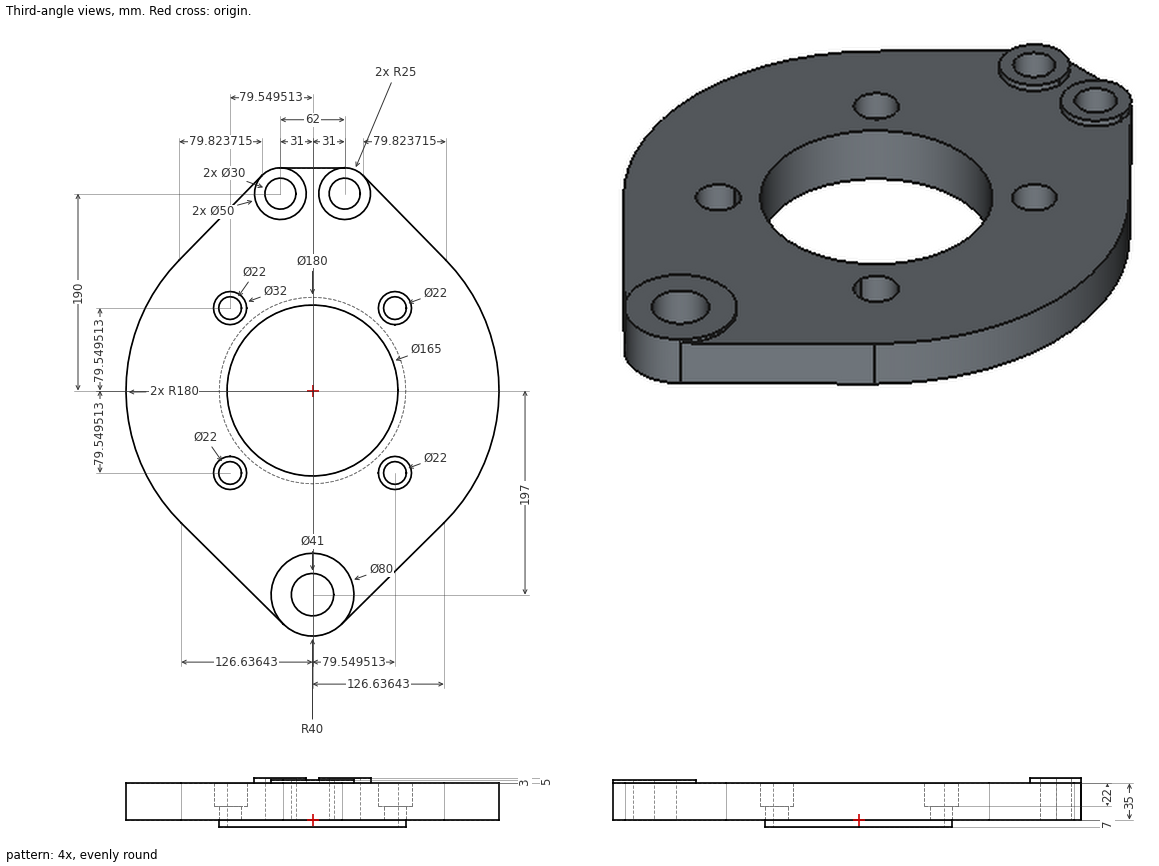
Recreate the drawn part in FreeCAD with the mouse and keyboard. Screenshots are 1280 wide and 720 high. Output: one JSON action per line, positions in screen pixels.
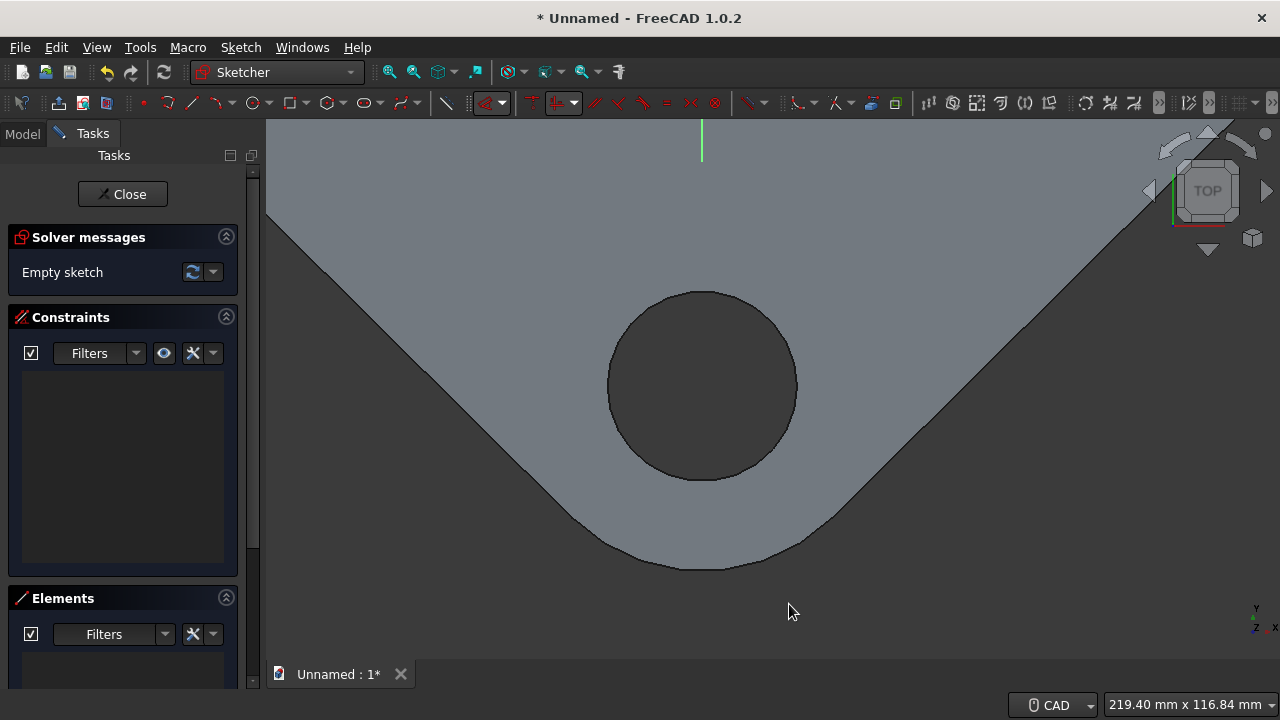
{"action": "key", "text": "g c"}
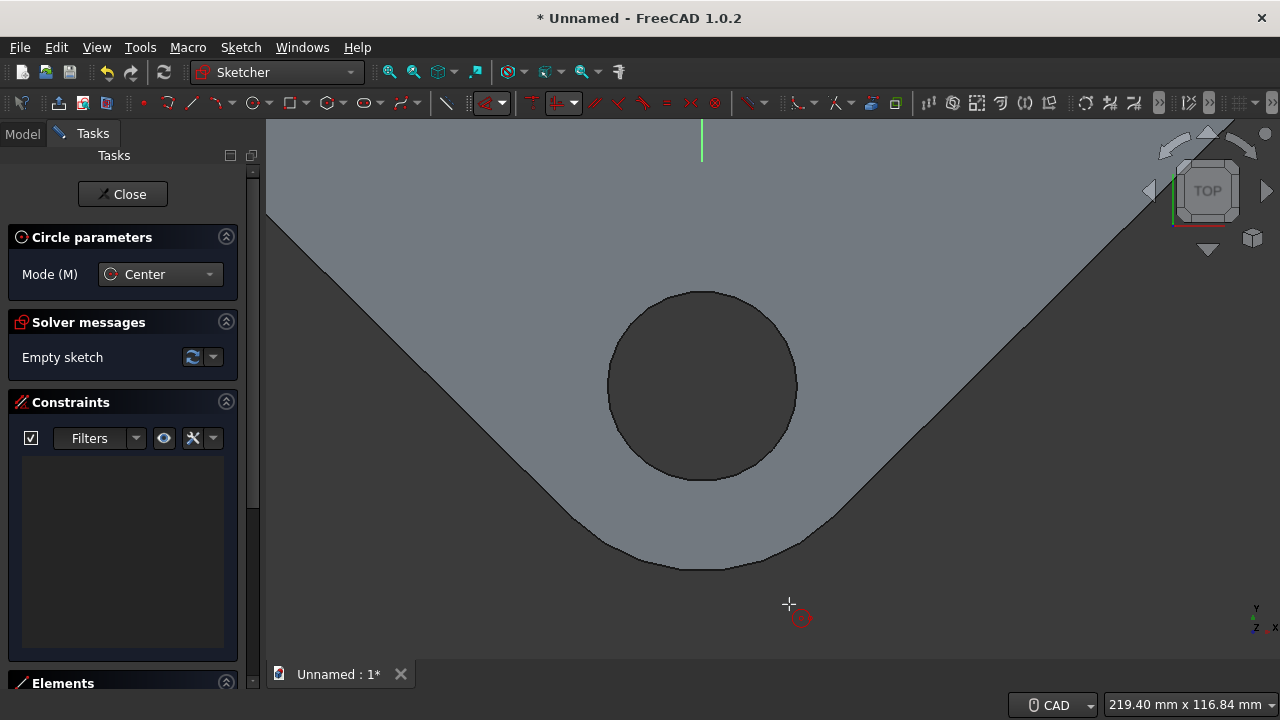
{"action": "left_click", "coordinate": [702, 386]}
{"action": "left_click", "coordinate": [833, 256]}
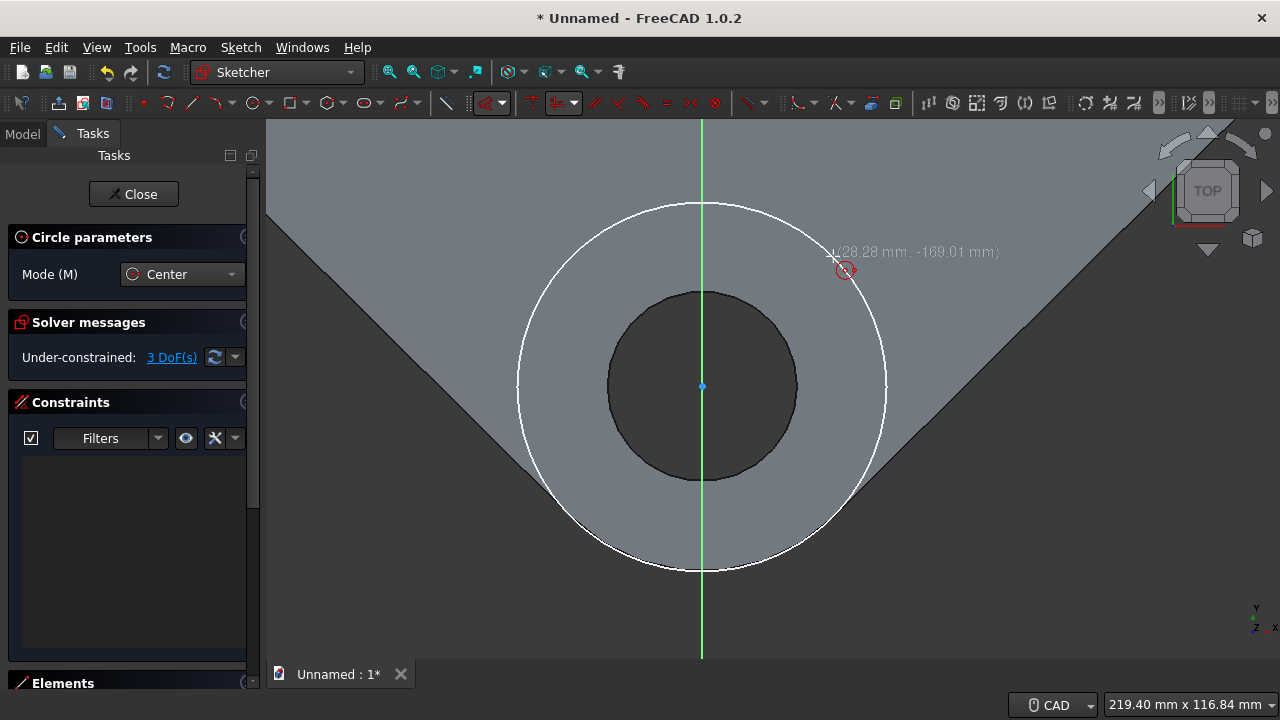
{"action": "left_click", "coordinate": [702, 387]}
{"action": "left_click", "coordinate": [769, 319]}
{"action": "key", "text": "Escape"}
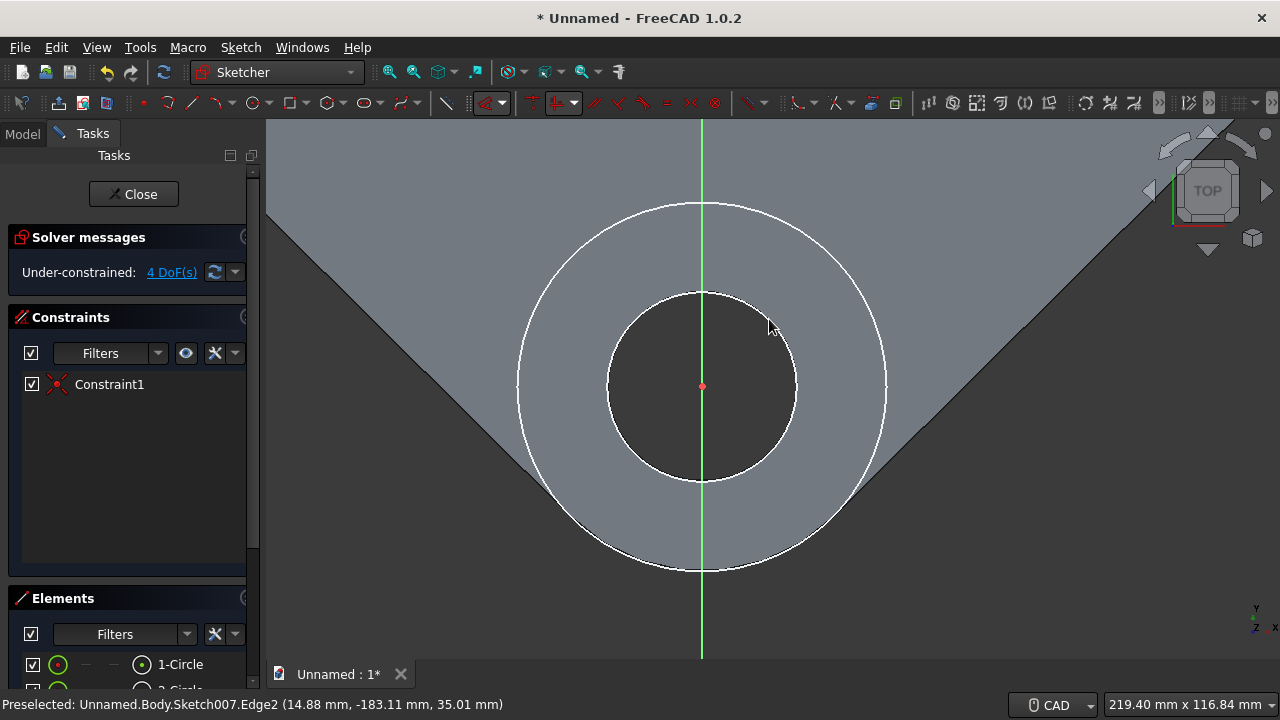
{"action": "left_click", "coordinate": [702, 387]}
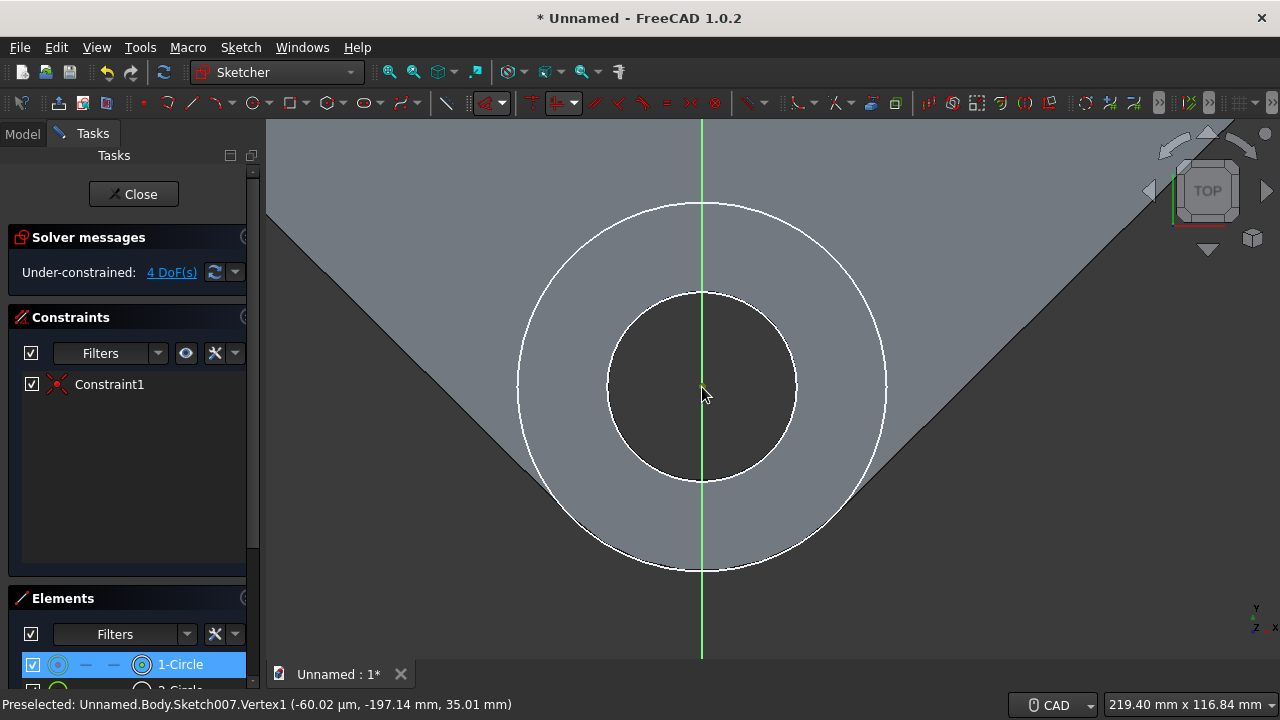
{"action": "left_click", "coordinate": [702, 527]}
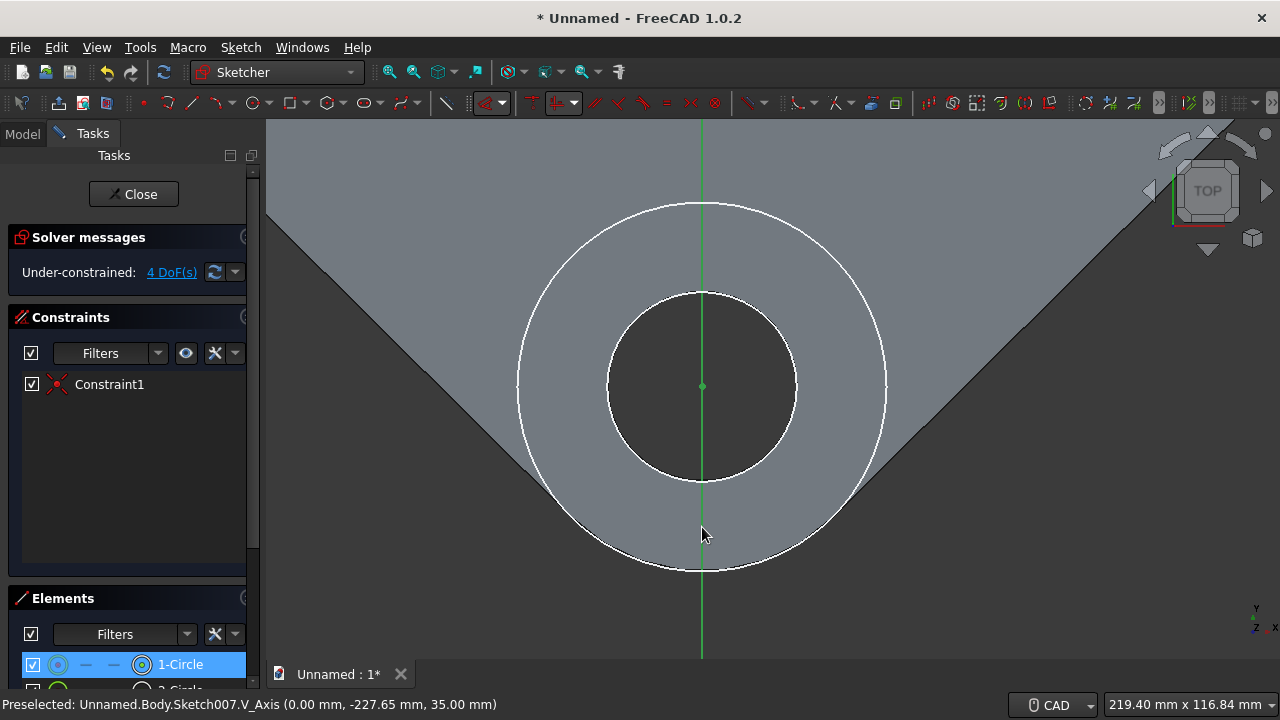
{"action": "key", "text": "c"}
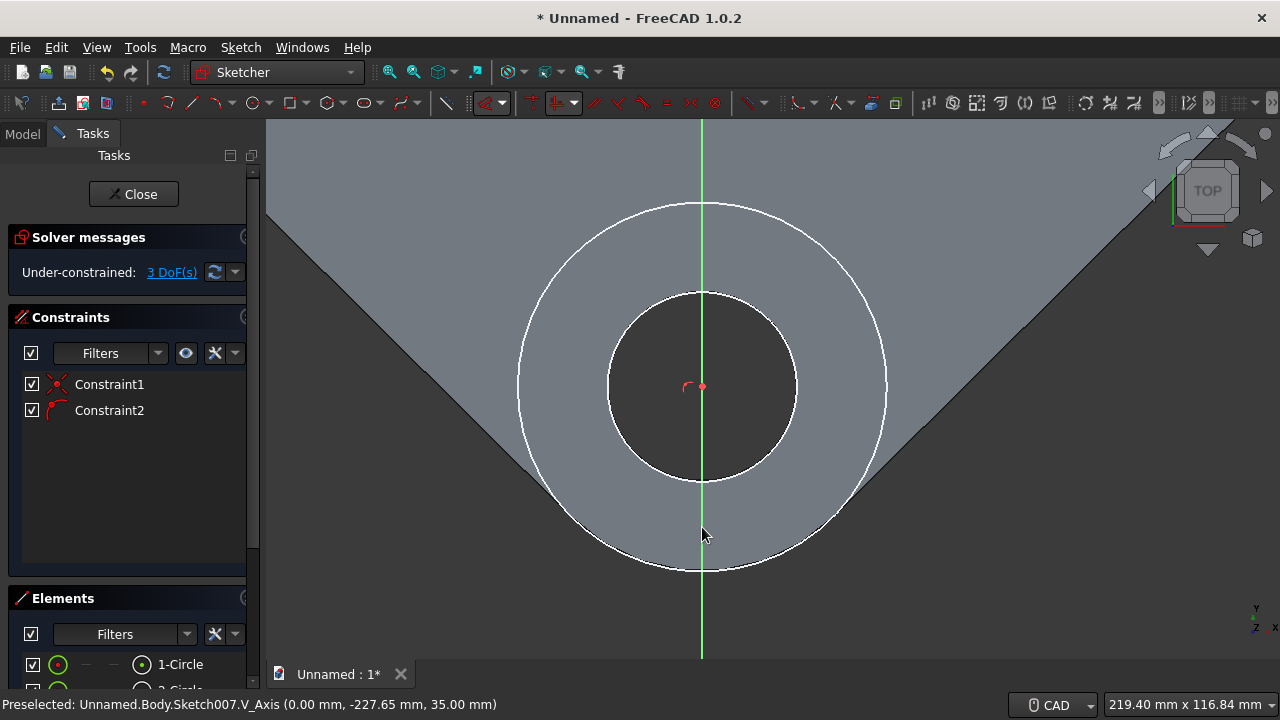
{"action": "left_click", "coordinate": [832, 256]}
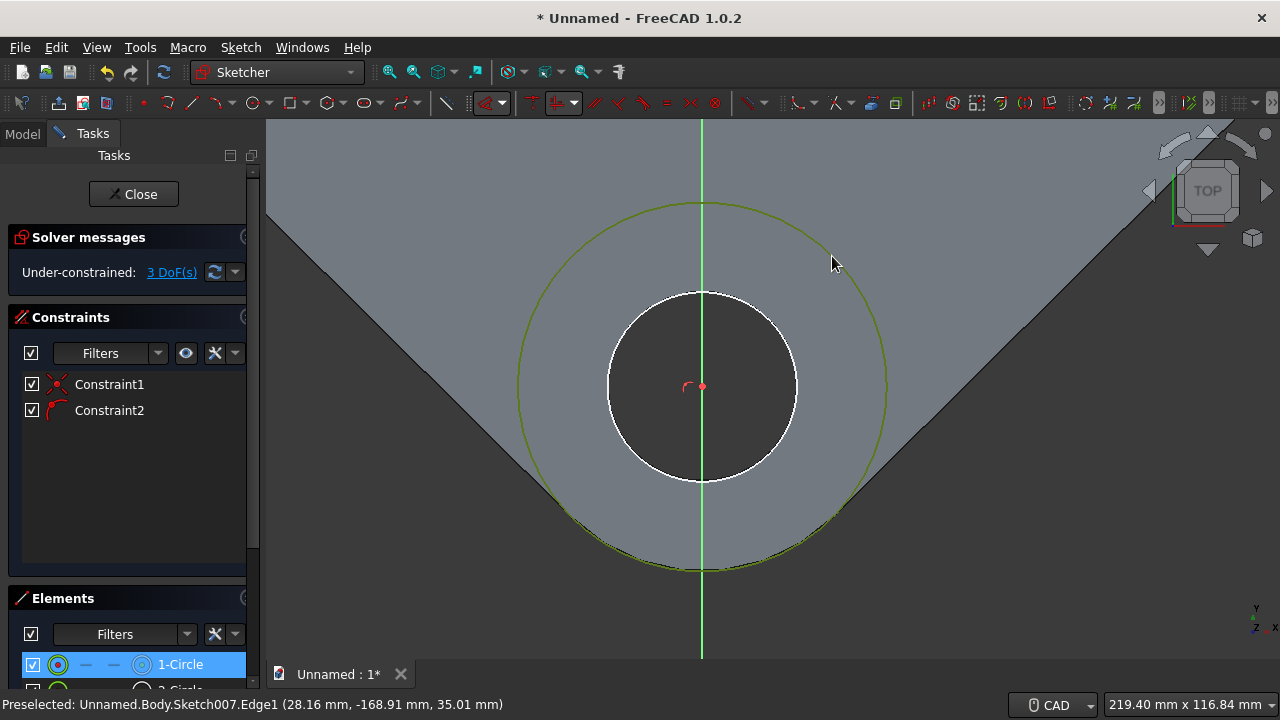
{"action": "left_click", "coordinate": [504, 104]}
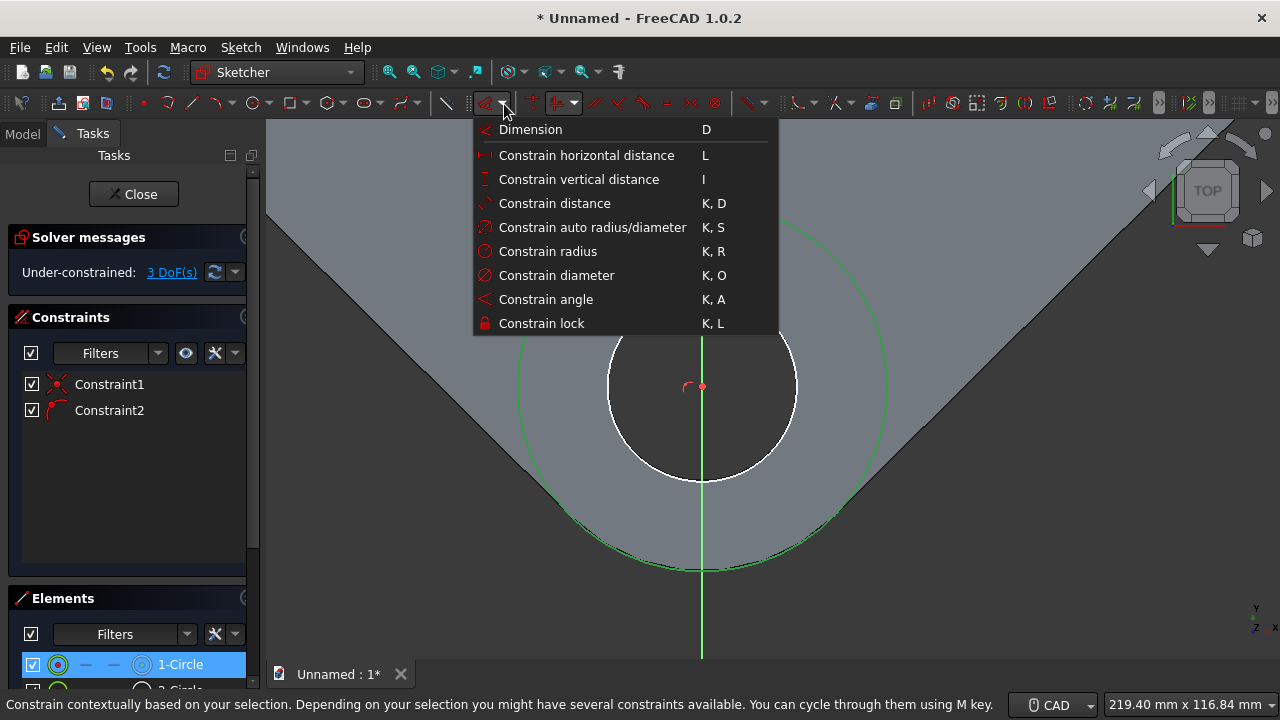
{"action": "left_click", "coordinate": [626, 275]}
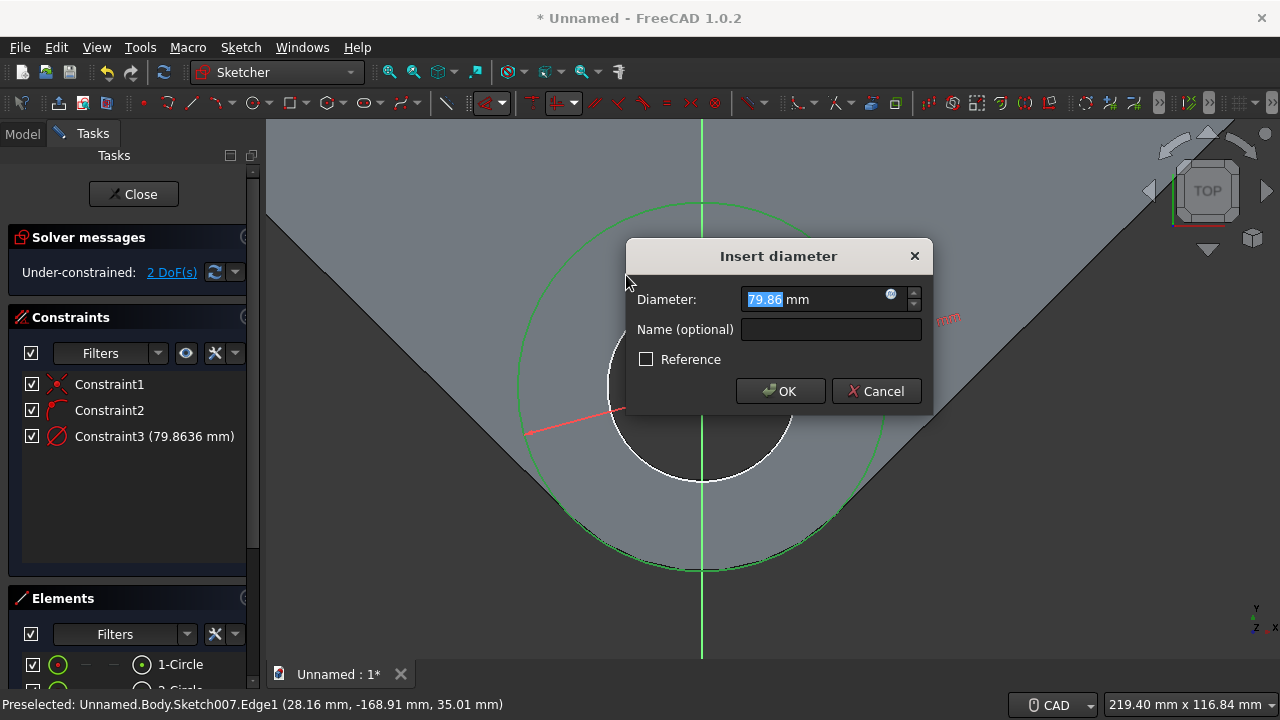
{"action": "type", "text": "80"}
{"action": "key", "text": "Return"}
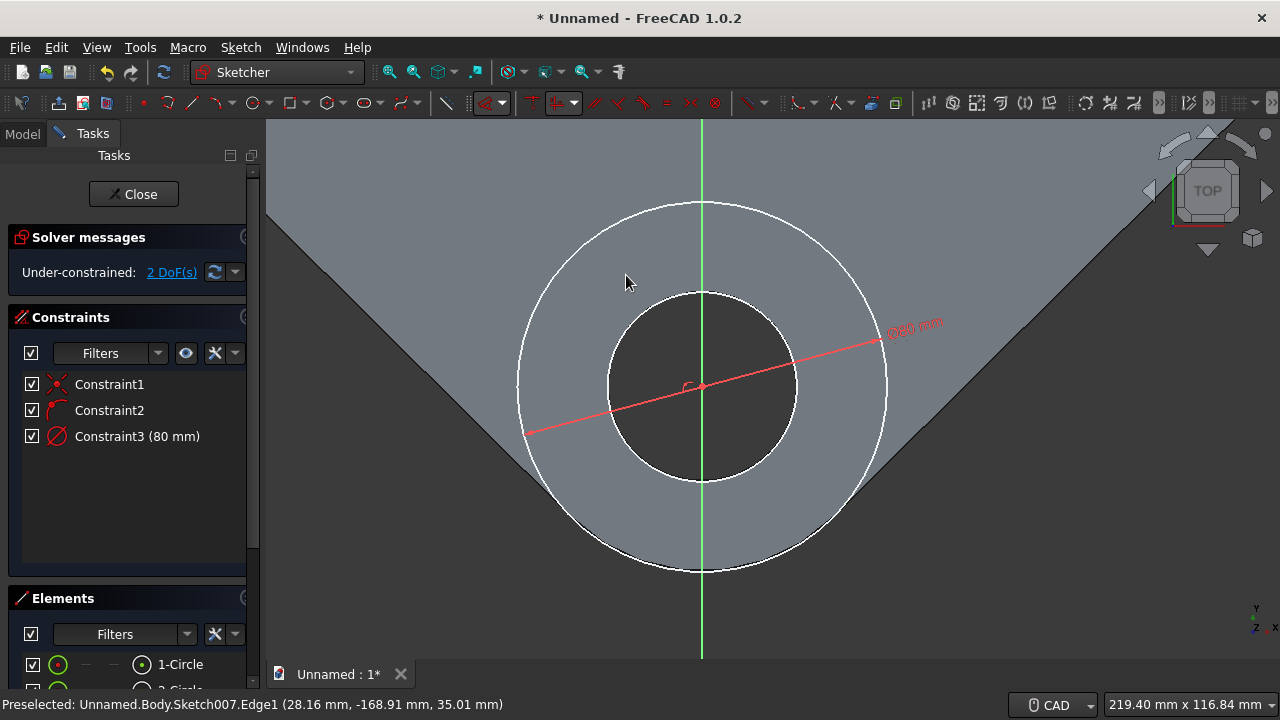
{"action": "left_click", "coordinate": [769, 320]}